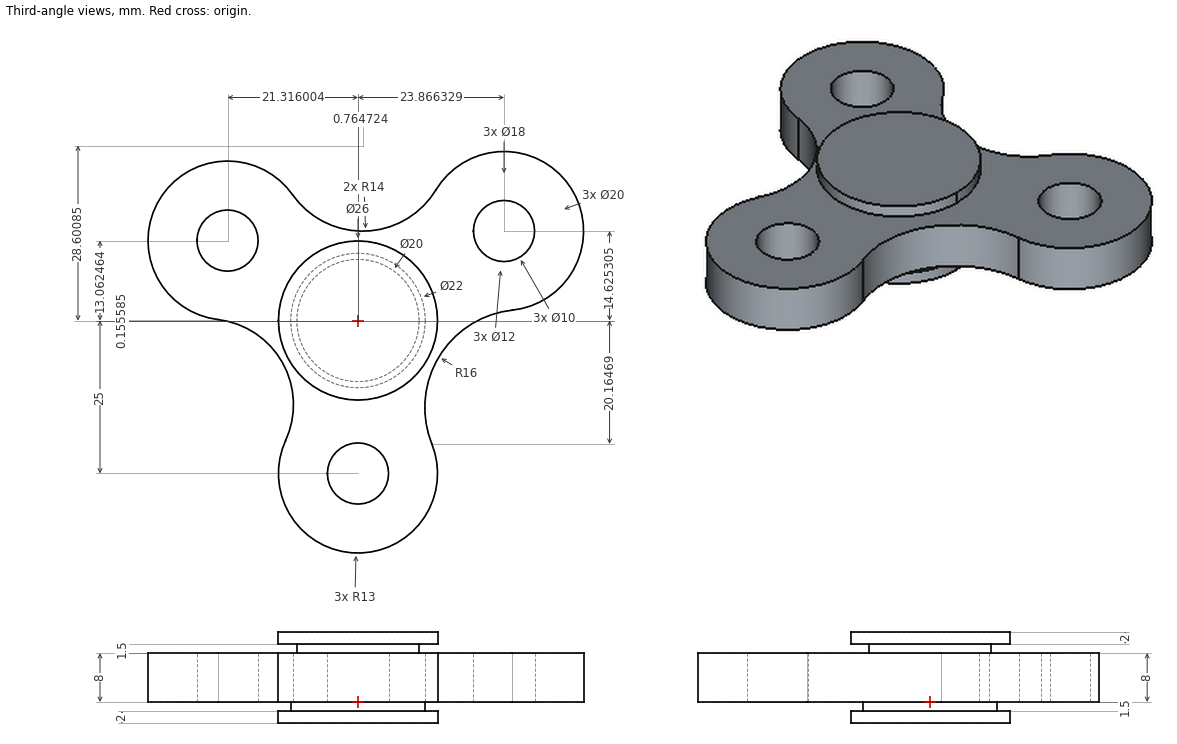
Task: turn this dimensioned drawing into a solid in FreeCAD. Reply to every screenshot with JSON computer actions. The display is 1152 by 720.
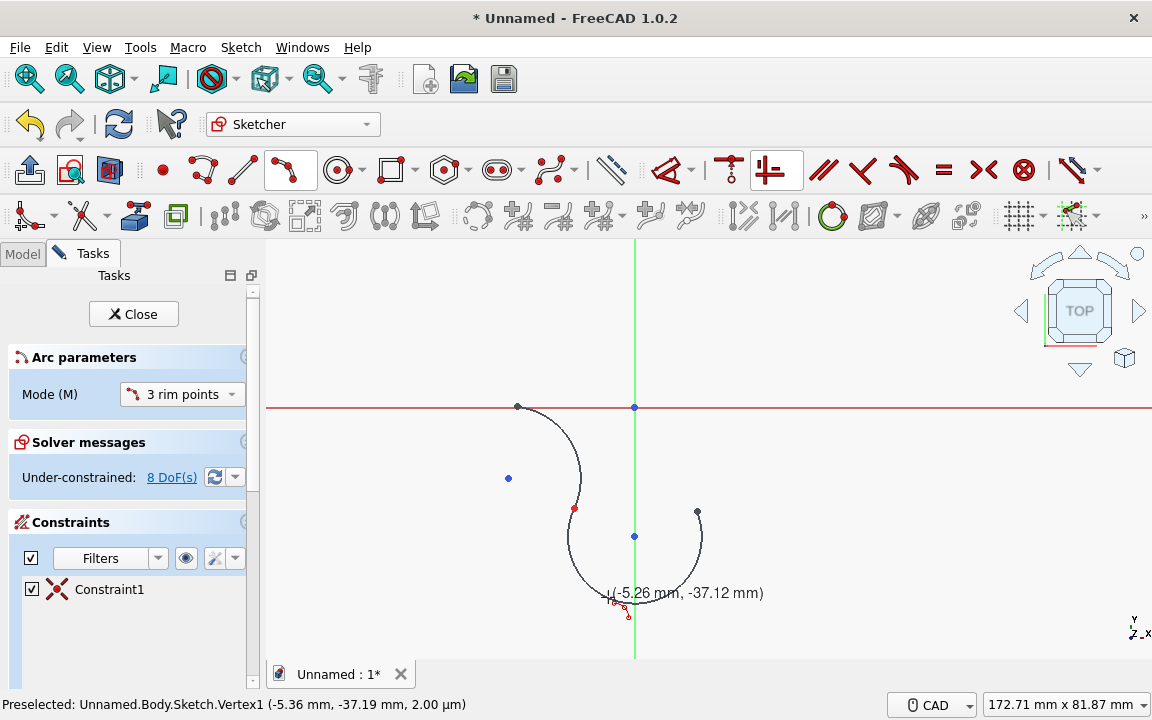
{"action": "left_click", "coordinate": [697, 512]}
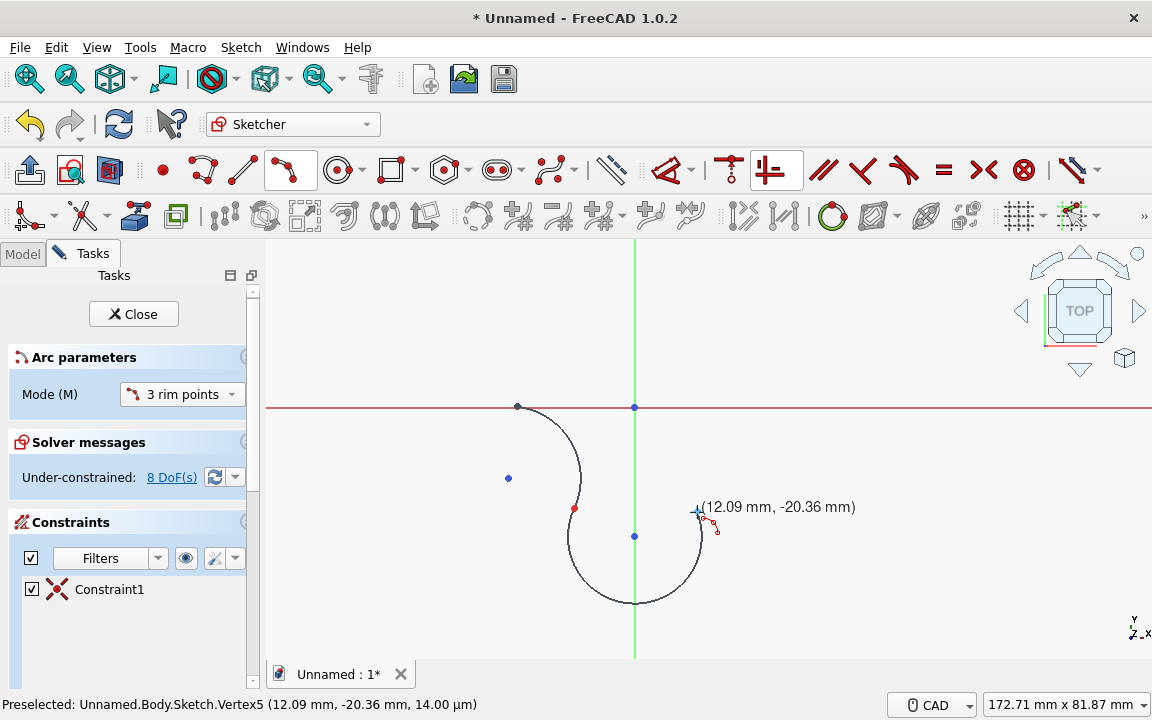
{"action": "scroll", "coordinate": [764, 399], "scroll_direction": "up", "scroll_amount": 4}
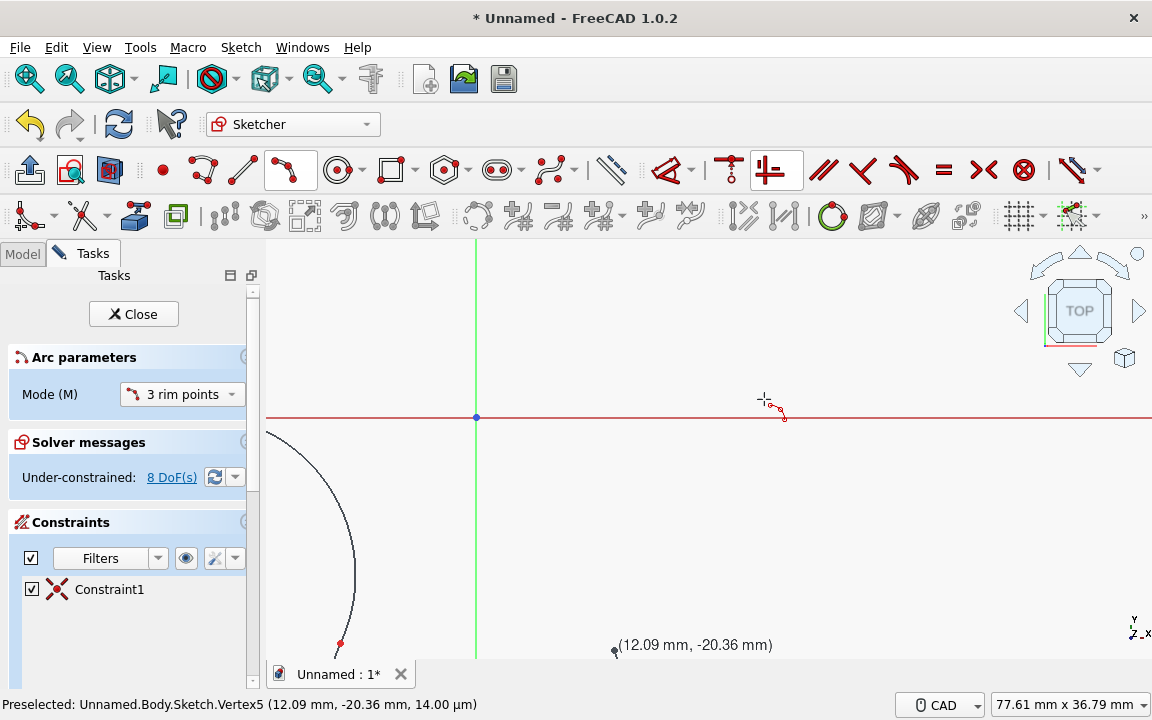
{"action": "left_click", "coordinate": [764, 398]}
{"action": "left_click", "coordinate": [627, 486]}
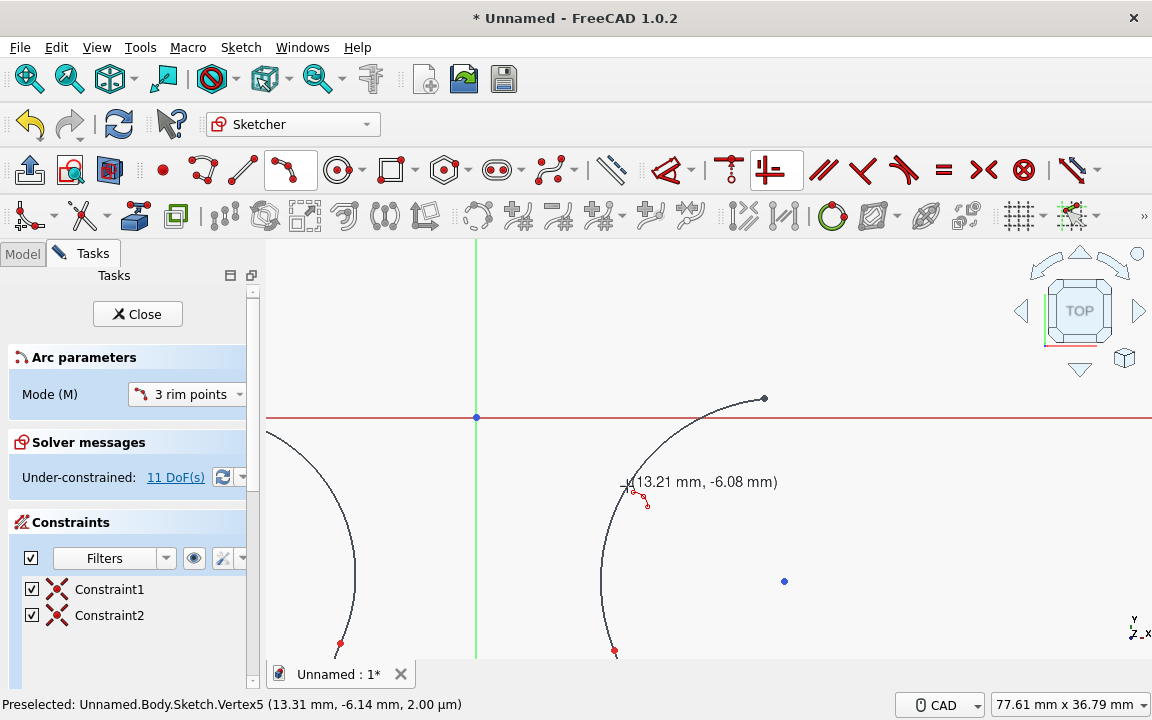
{"action": "left_click", "coordinate": [764, 399]}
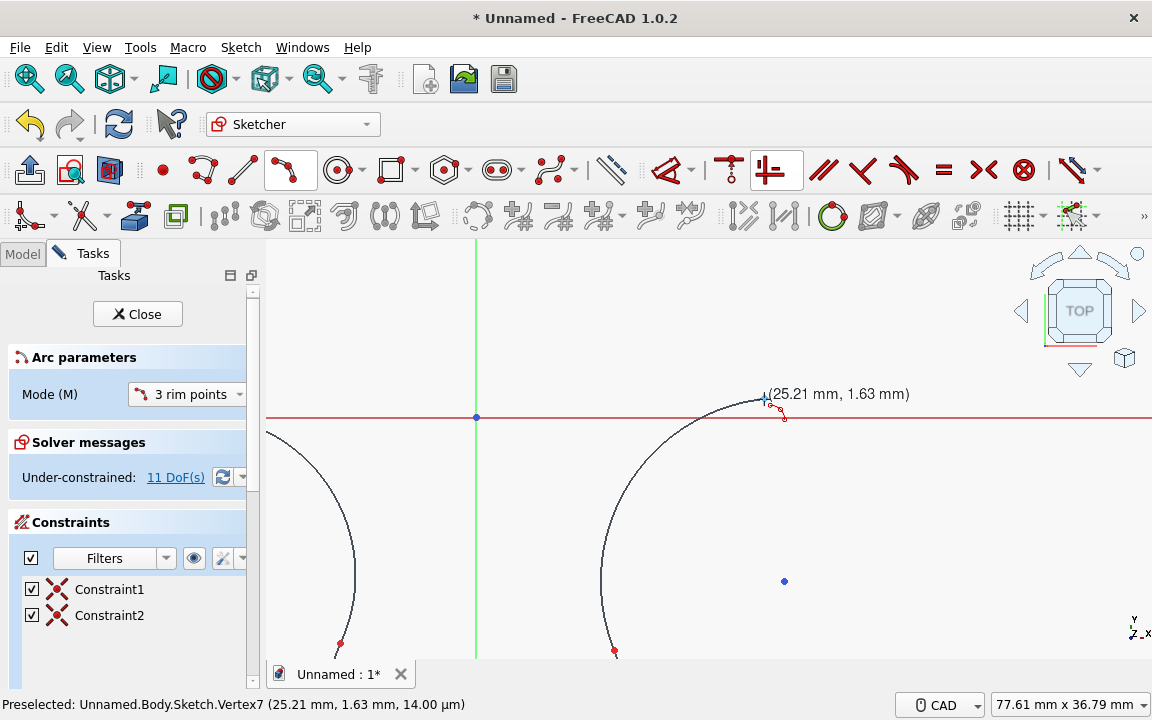
{"action": "scroll", "coordinate": [728, 413], "scroll_direction": "down", "scroll_amount": 5}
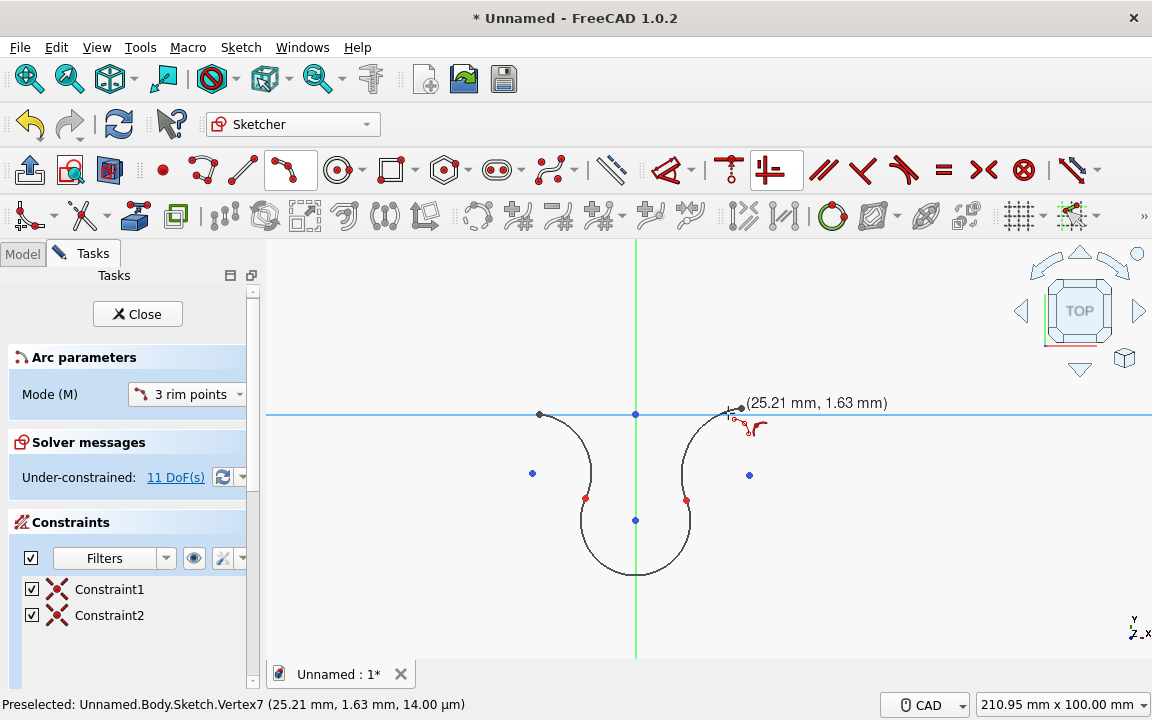
{"action": "left_click", "coordinate": [689, 325]}
{"action": "left_click", "coordinate": [782, 324]}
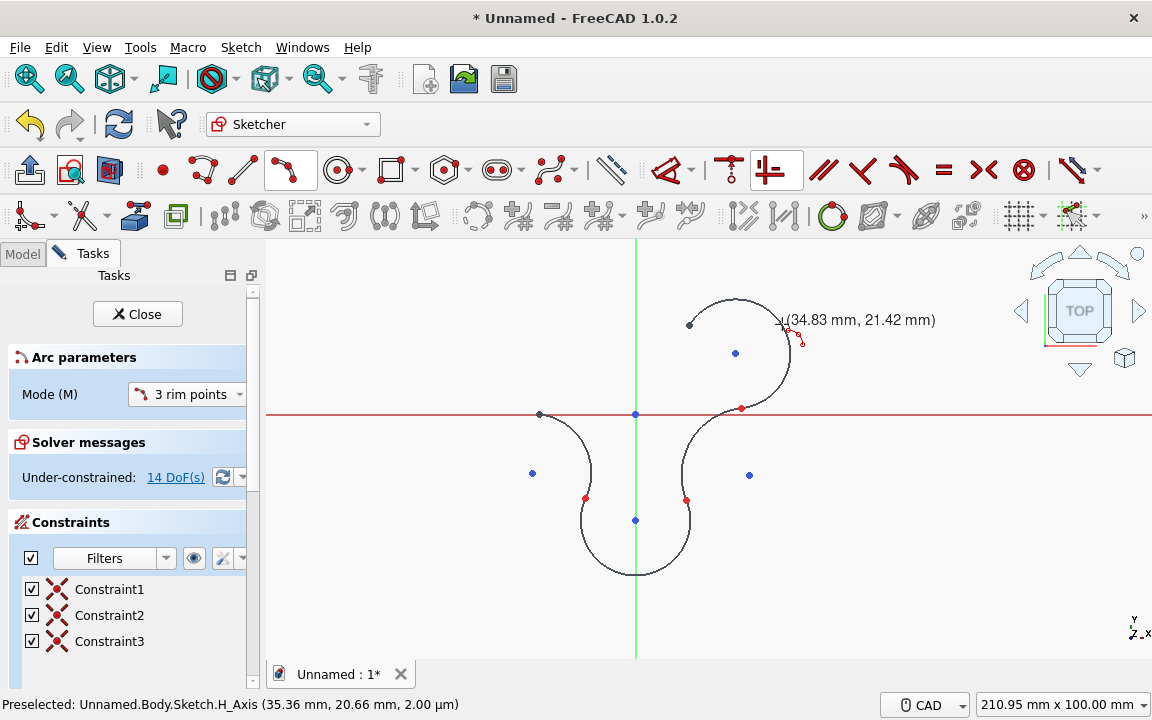
{"action": "left_click", "coordinate": [689, 326]}
{"action": "left_click", "coordinate": [591, 329]}
{"action": "left_click", "coordinate": [618, 350]}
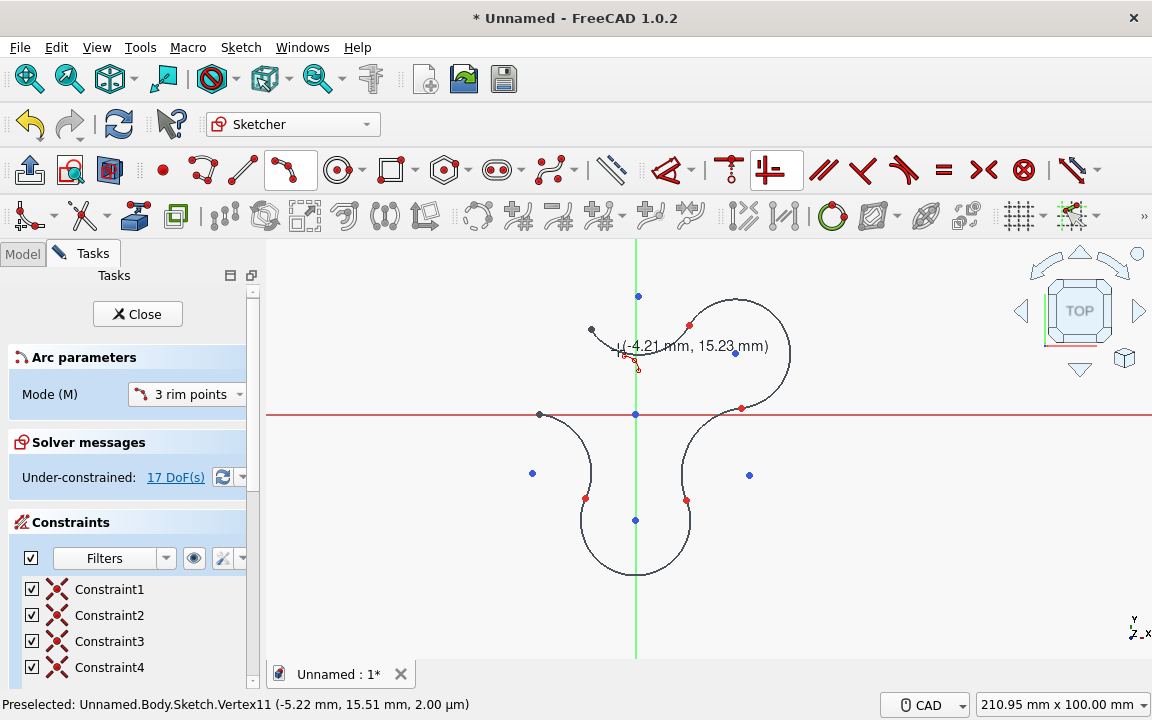
{"action": "left_click", "coordinate": [591, 330]}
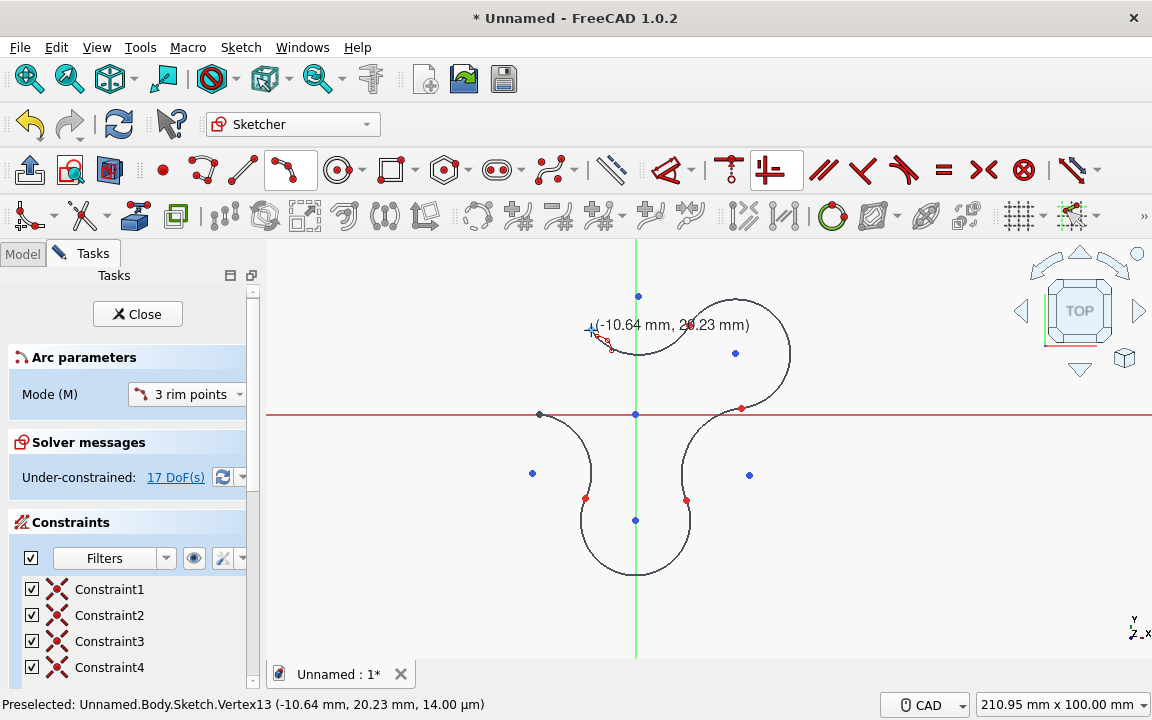
{"action": "scroll", "coordinate": [540, 414], "scroll_direction": "up", "scroll_amount": 16}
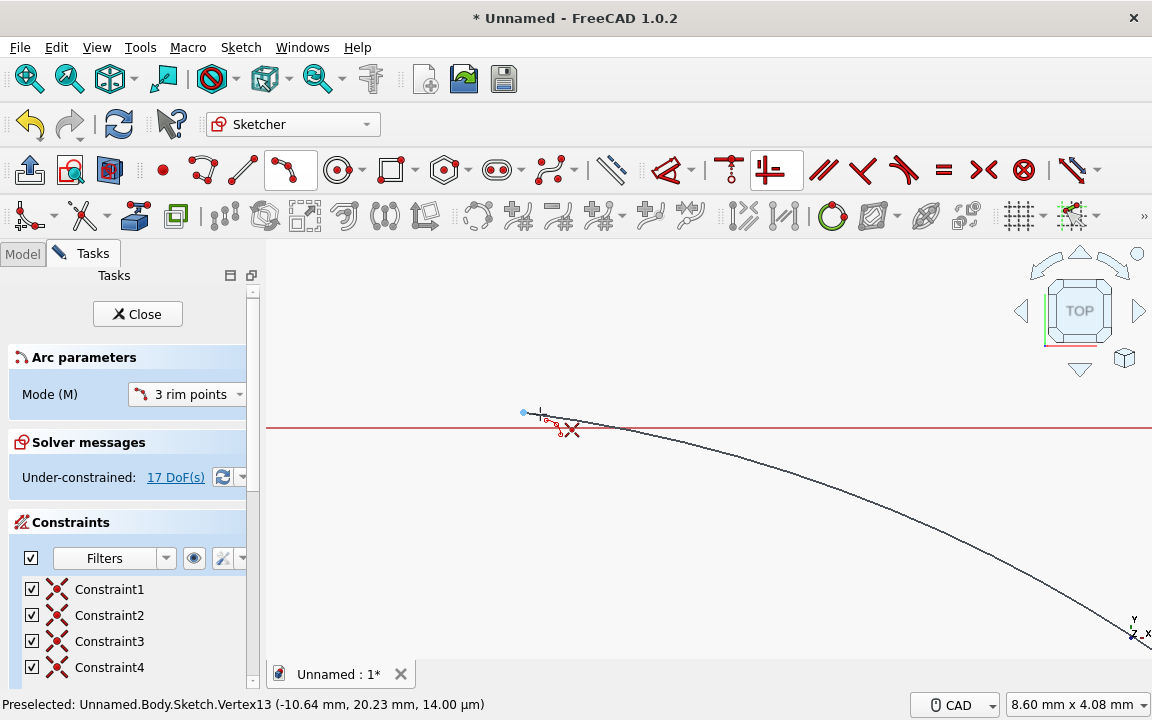
{"action": "left_click", "coordinate": [524, 413]}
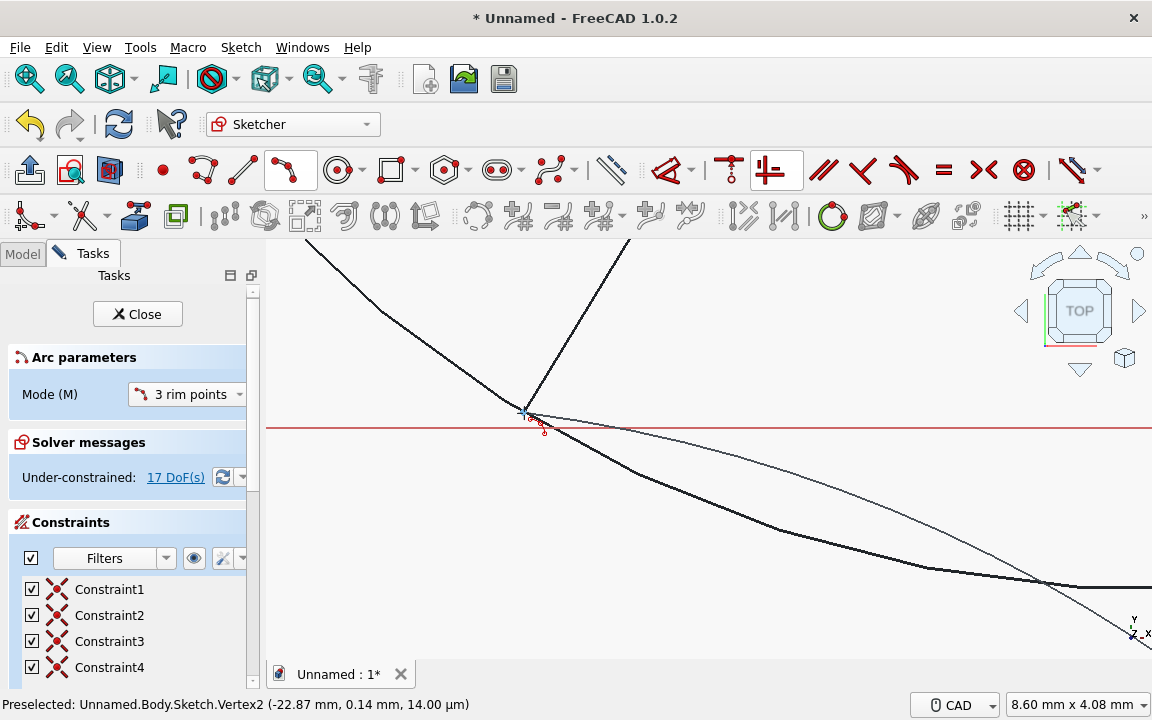
{"action": "scroll", "coordinate": [517, 406], "scroll_direction": "down", "scroll_amount": 15}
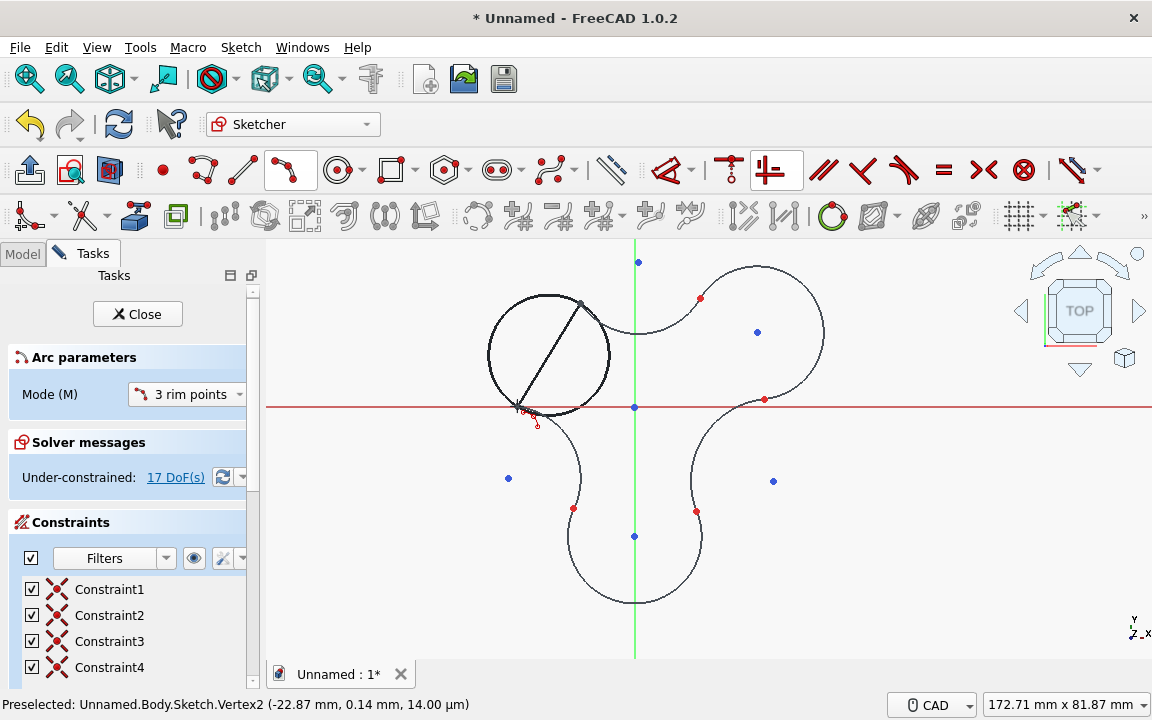
{"action": "left_click", "coordinate": [468, 306]}
{"action": "key", "text": "Escape"}